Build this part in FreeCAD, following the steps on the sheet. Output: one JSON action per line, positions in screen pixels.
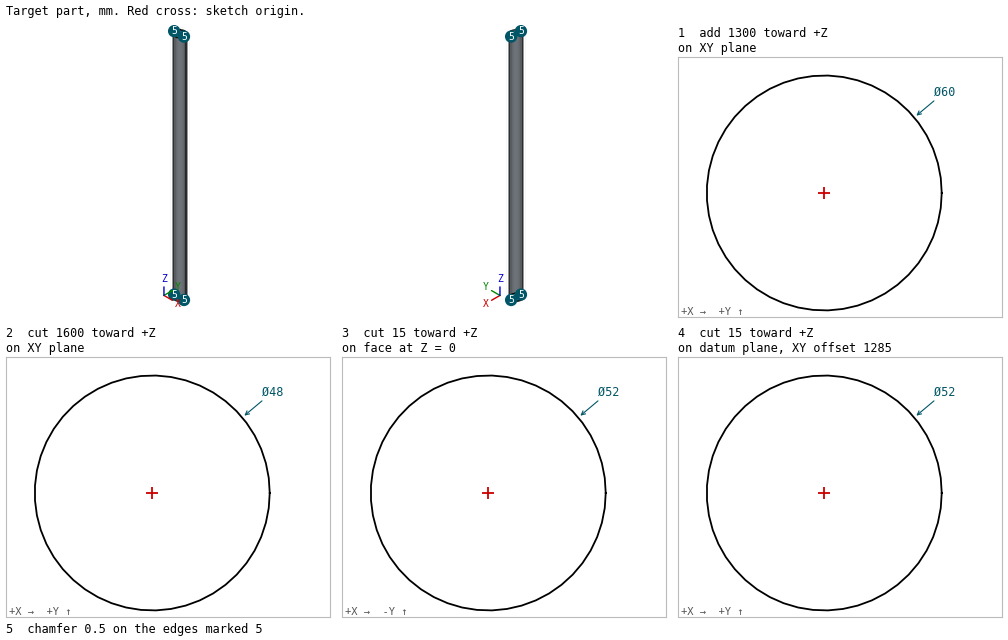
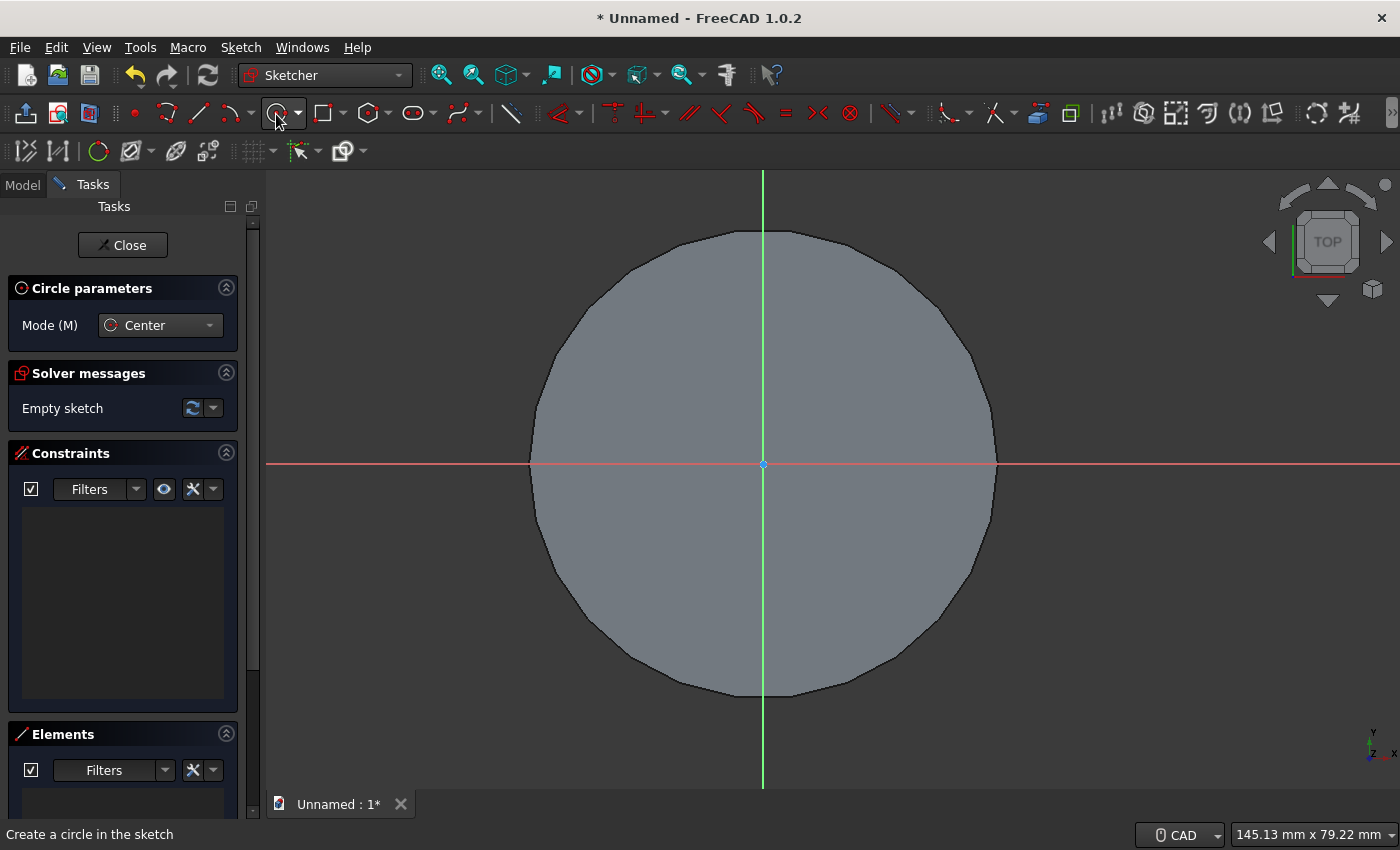
{"action": "left_click", "coordinate": [763, 464]}
{"action": "mouse_move", "coordinate": [896, 331]}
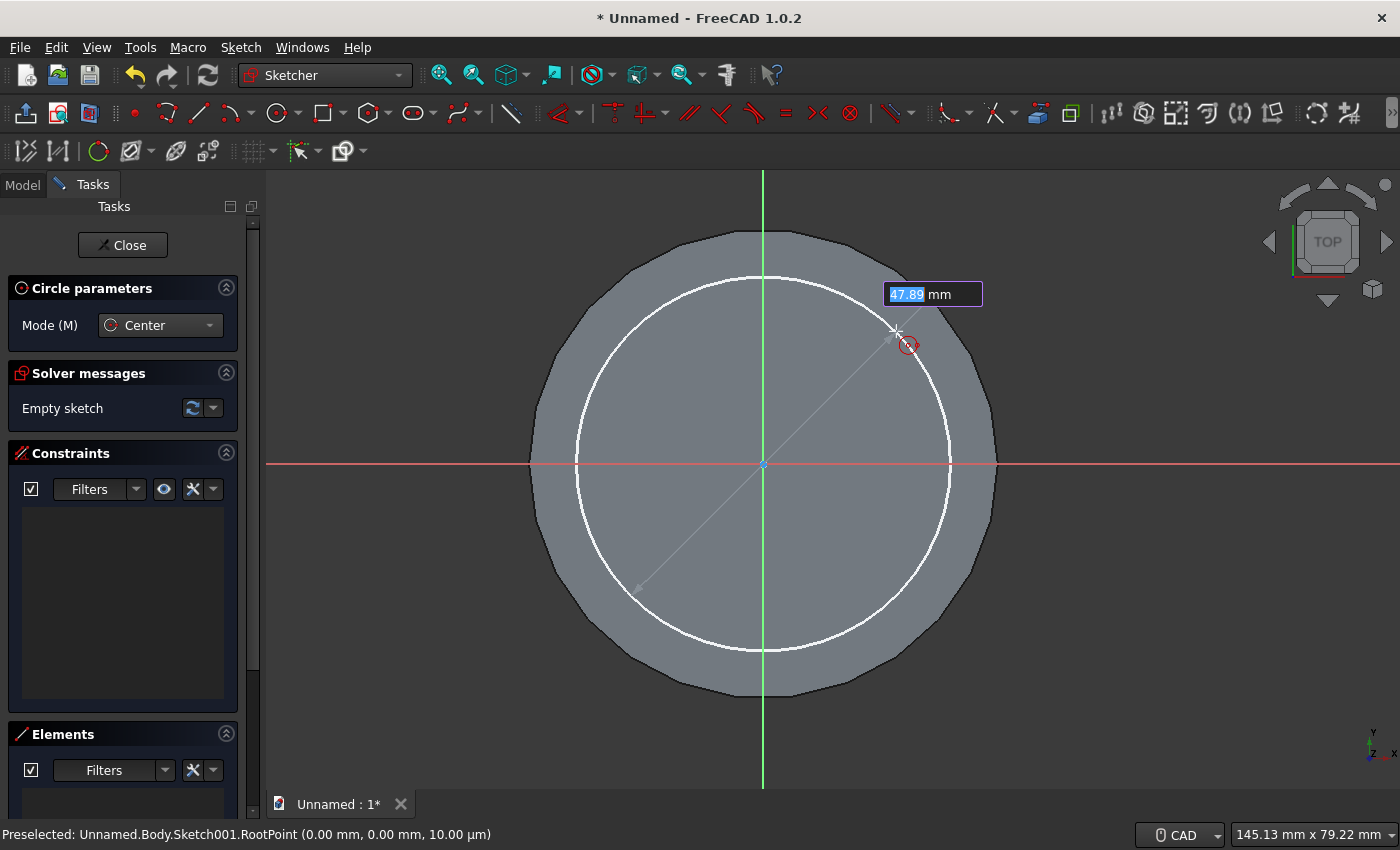
{"action": "type", "text": "48"}
{"action": "key", "text": "Return"}
{"action": "key", "text": "Escape"}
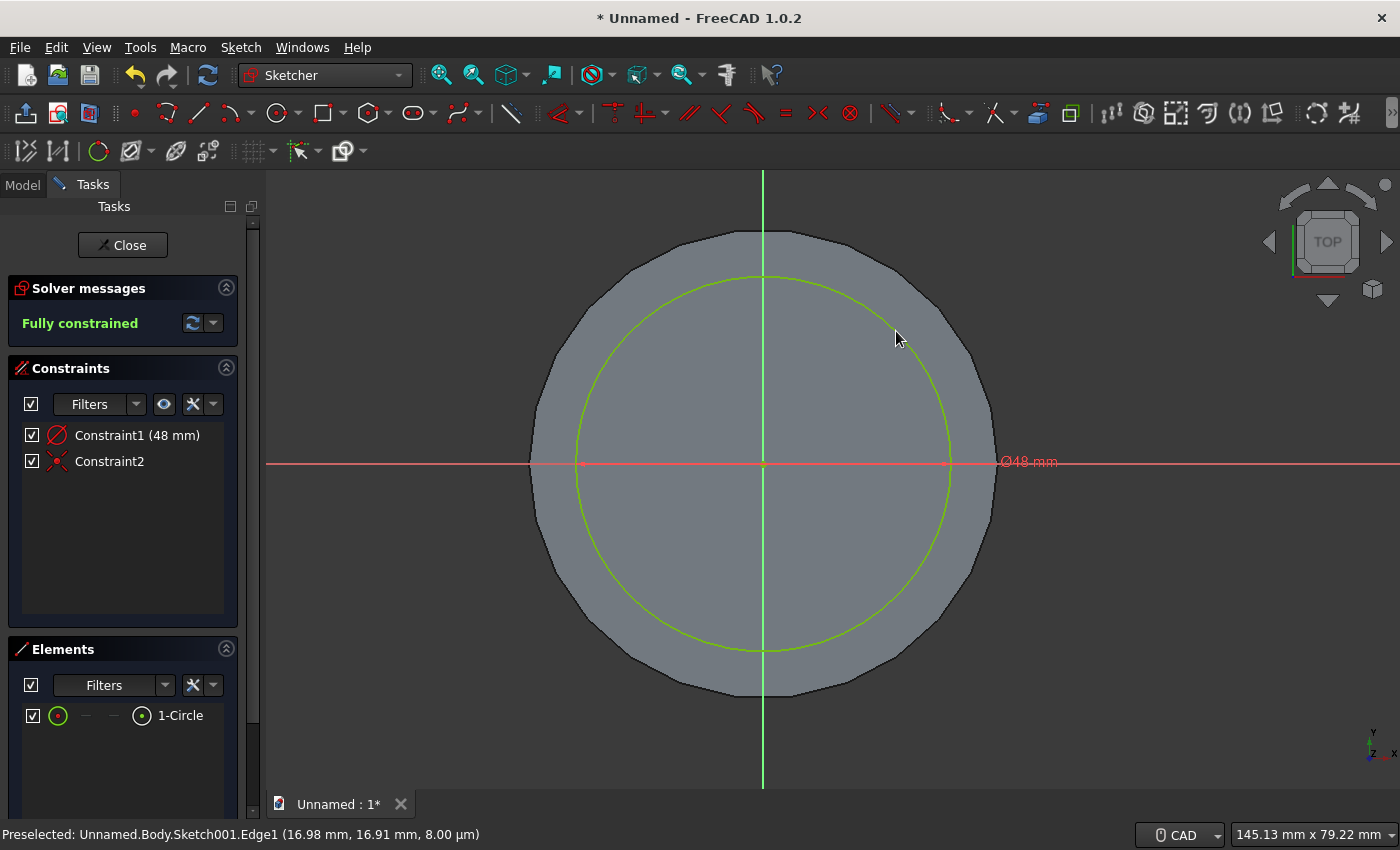
{"action": "left_click", "coordinate": [123, 245]}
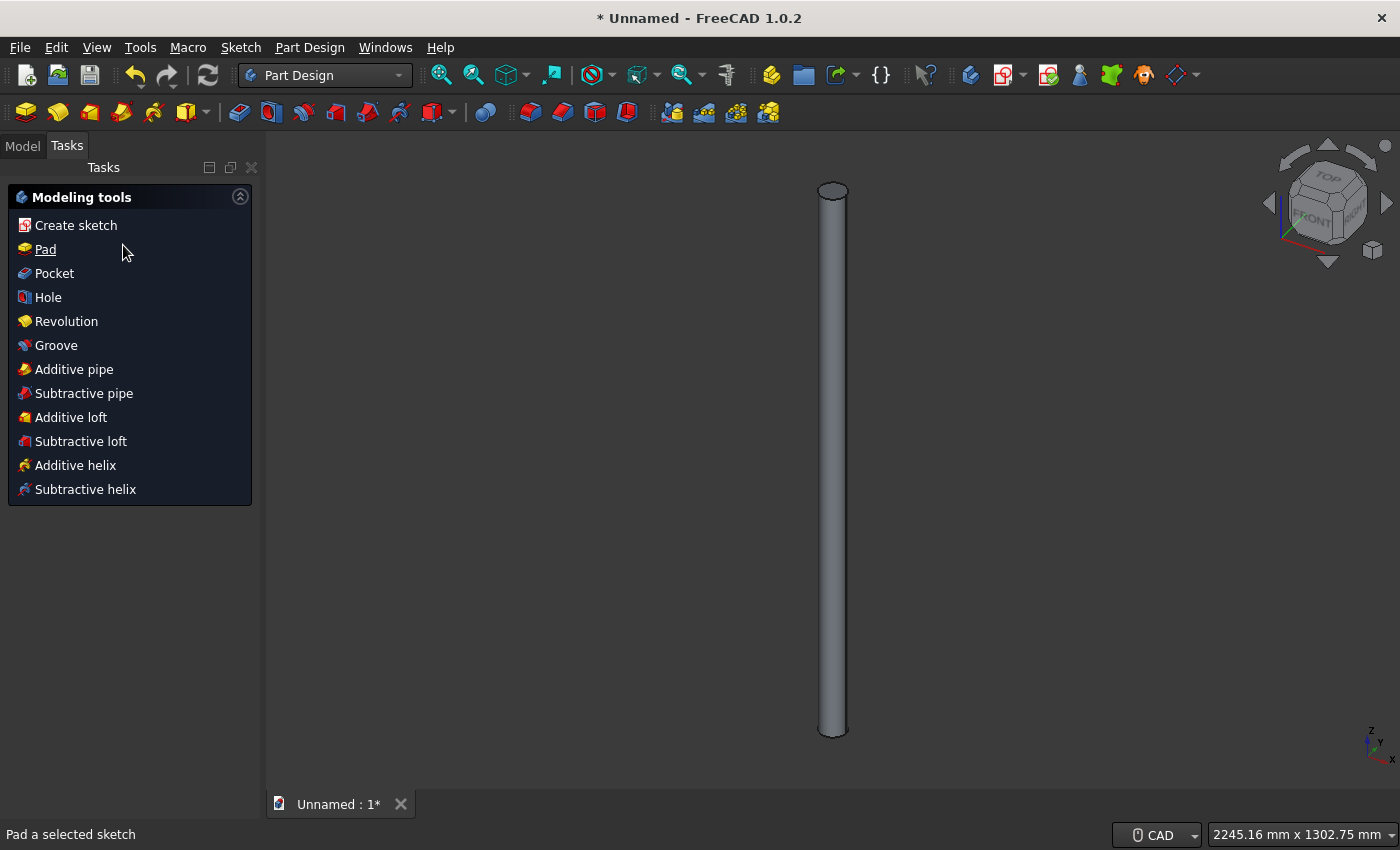
{"action": "left_click", "coordinate": [240, 112]}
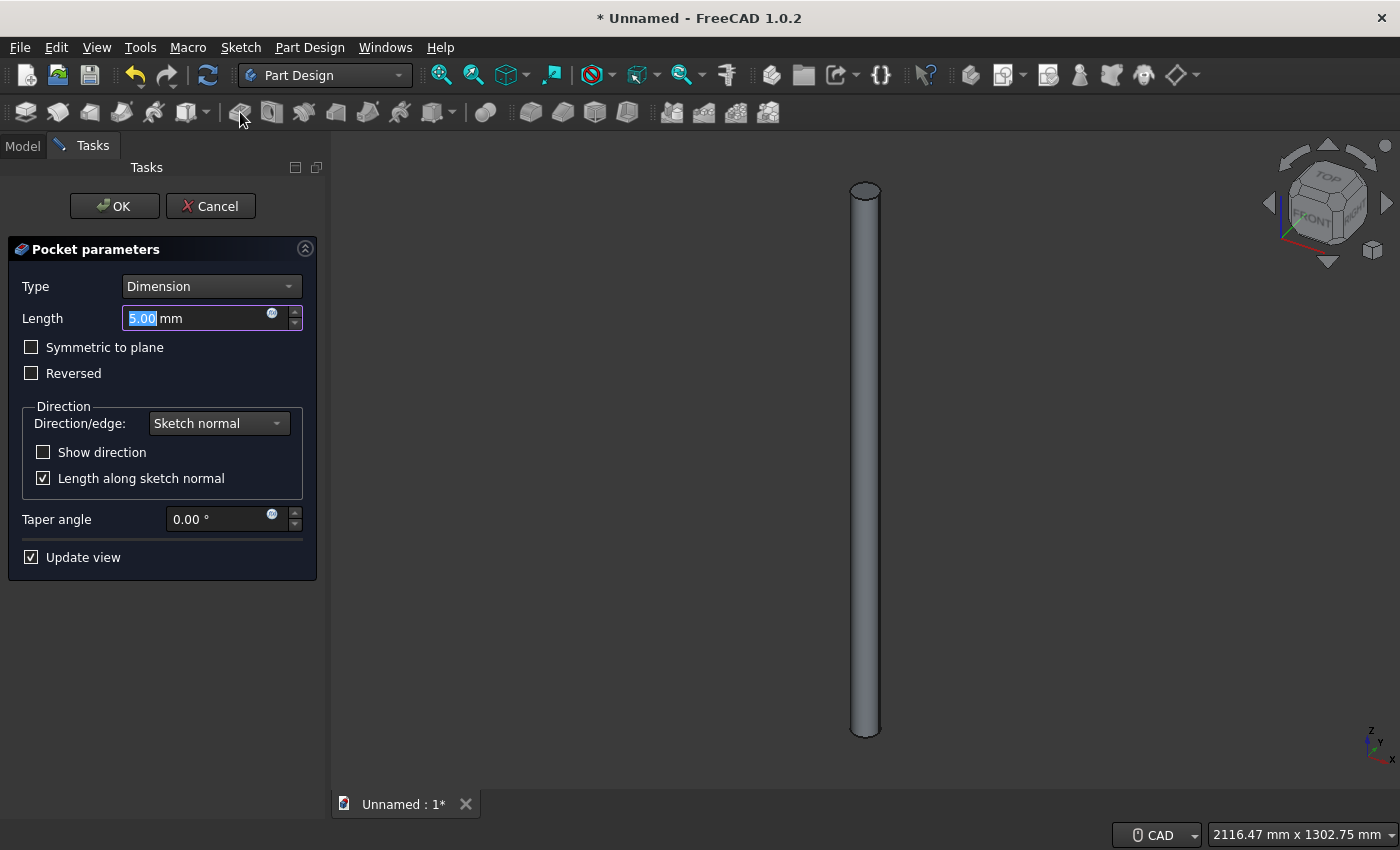
{"action": "type", "text": "1600"}
{"action": "key", "text": "Tab"}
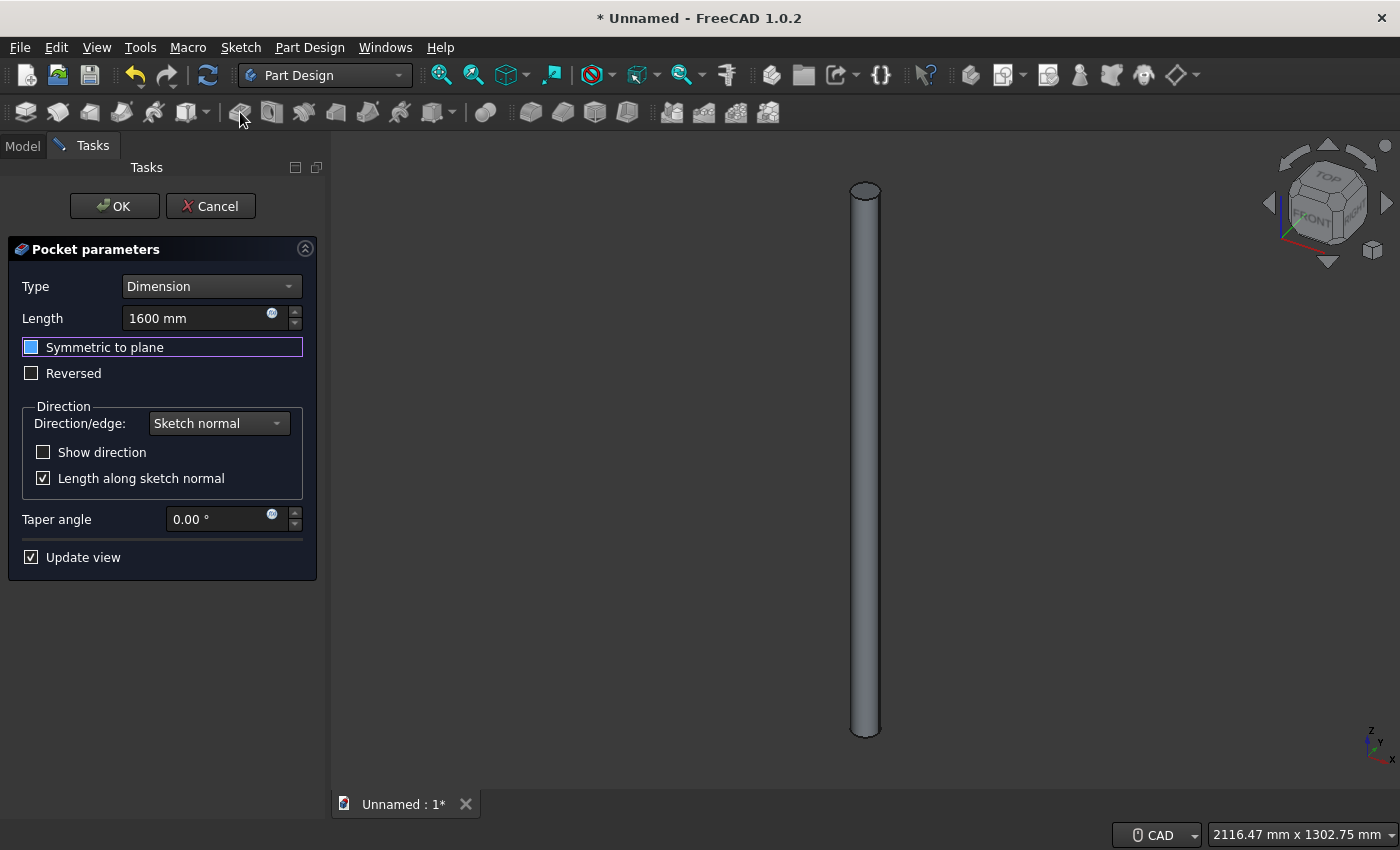
{"action": "left_click", "coordinate": [30, 373]}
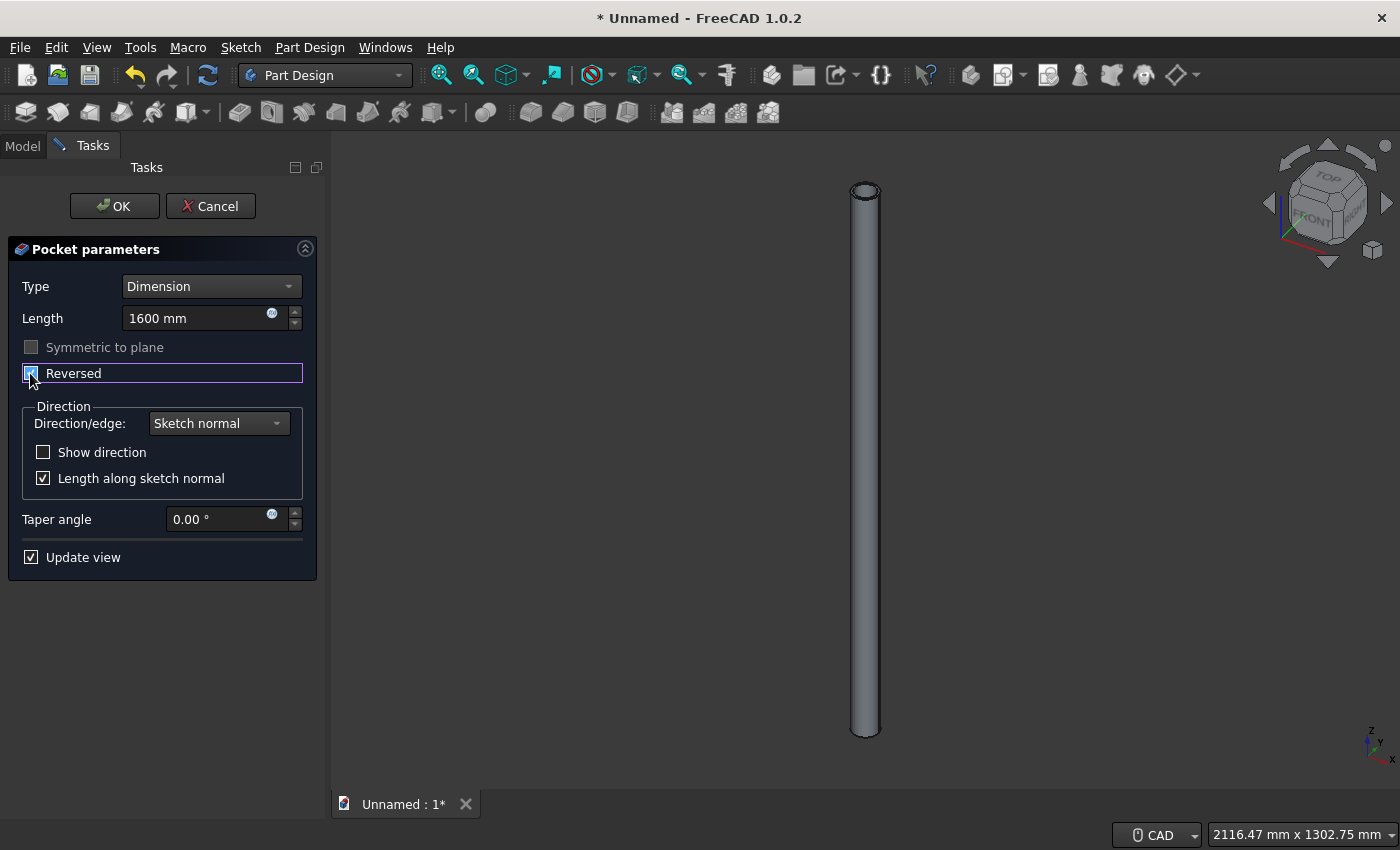
{"action": "left_click", "coordinate": [115, 206]}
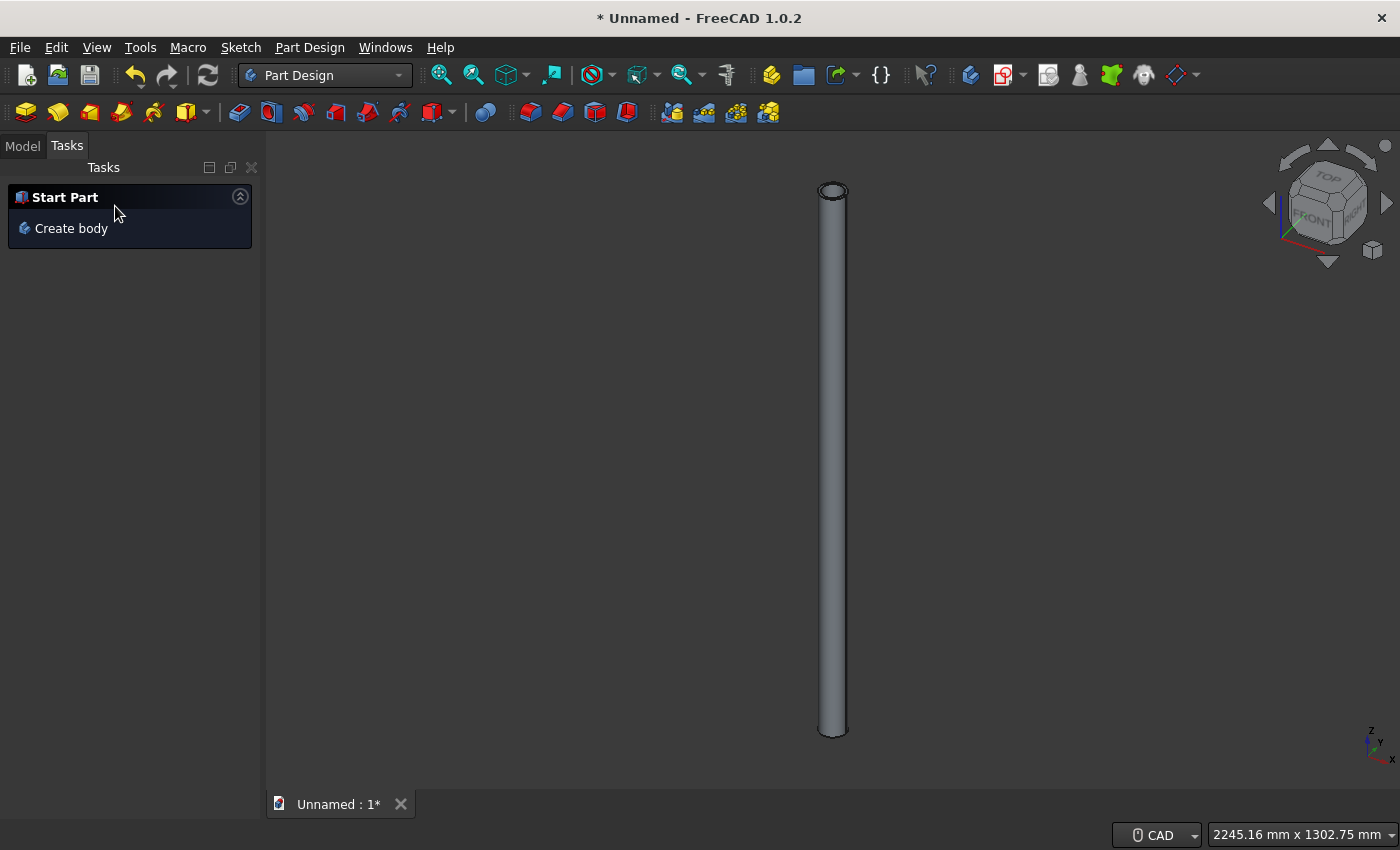
{"action": "key", "text": "5"}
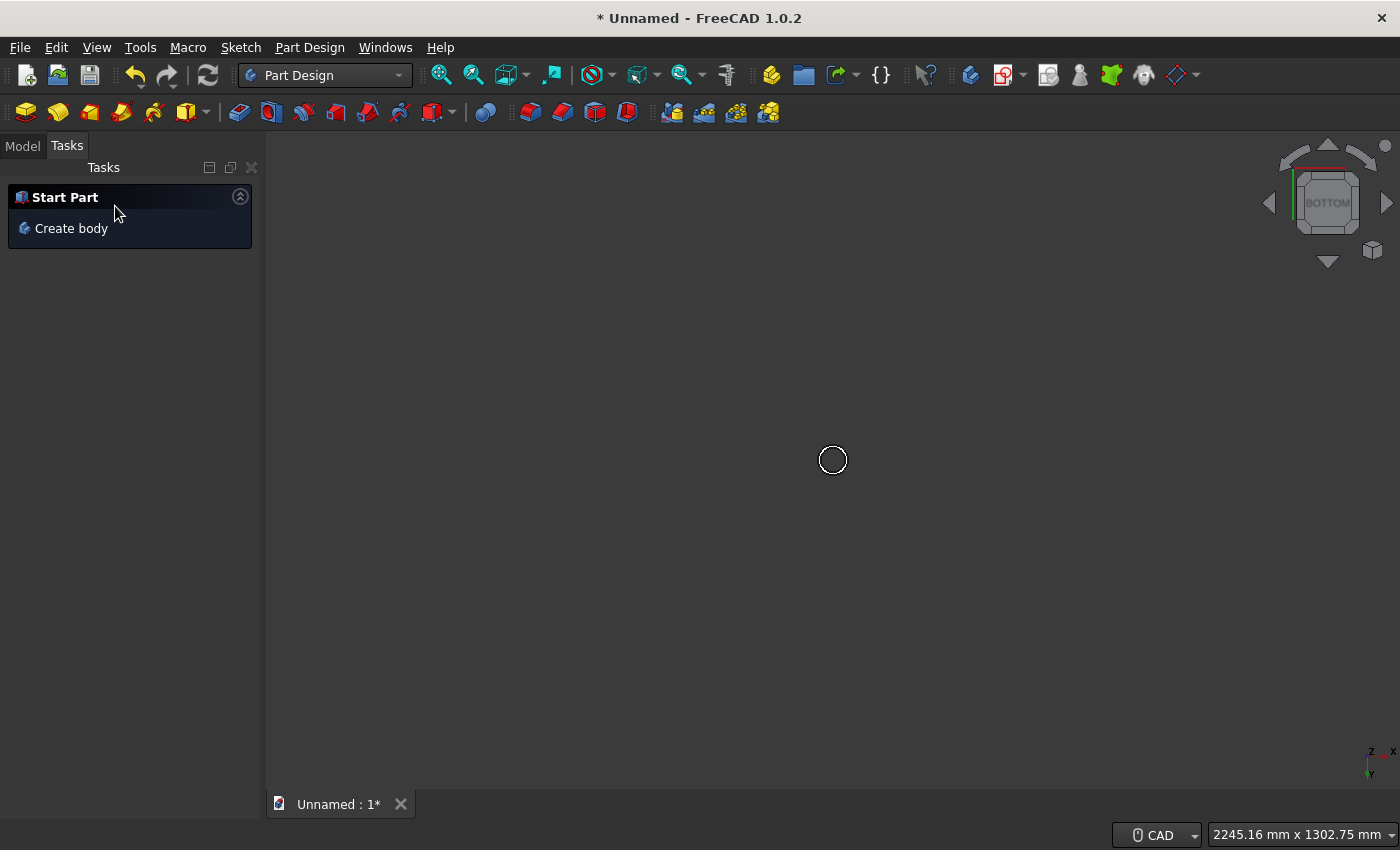
{"action": "left_click", "coordinate": [442, 76]}